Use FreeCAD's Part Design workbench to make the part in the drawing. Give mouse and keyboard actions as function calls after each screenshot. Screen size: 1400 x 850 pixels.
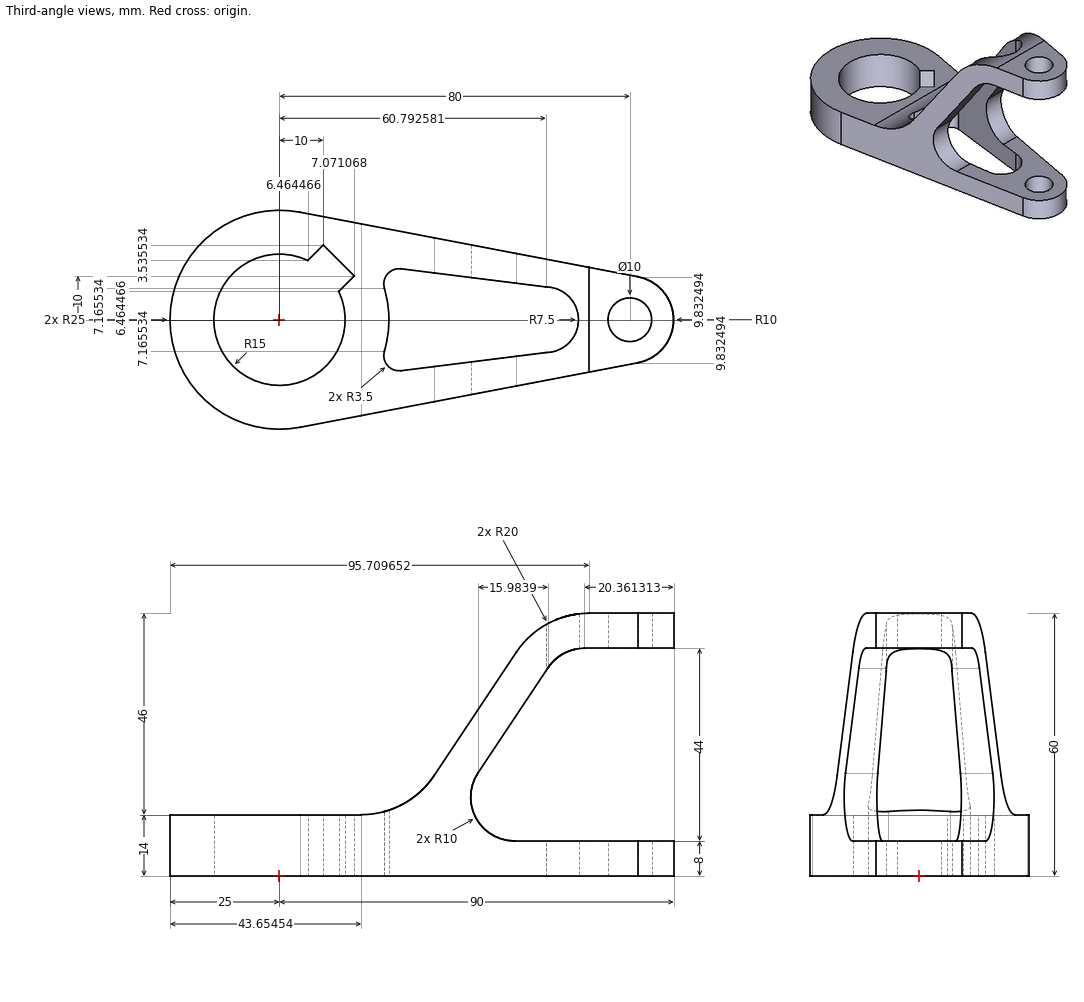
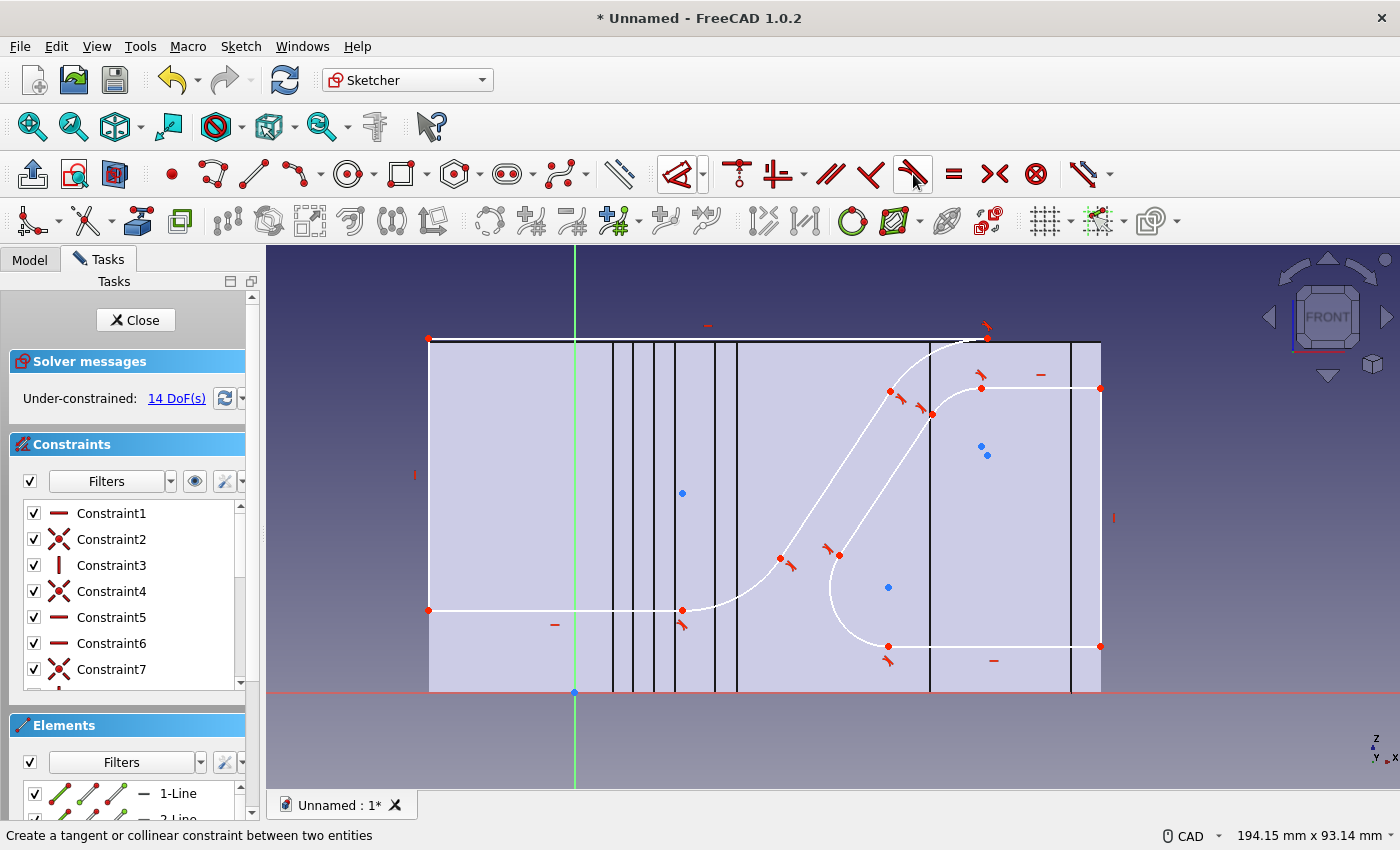
click(914, 366)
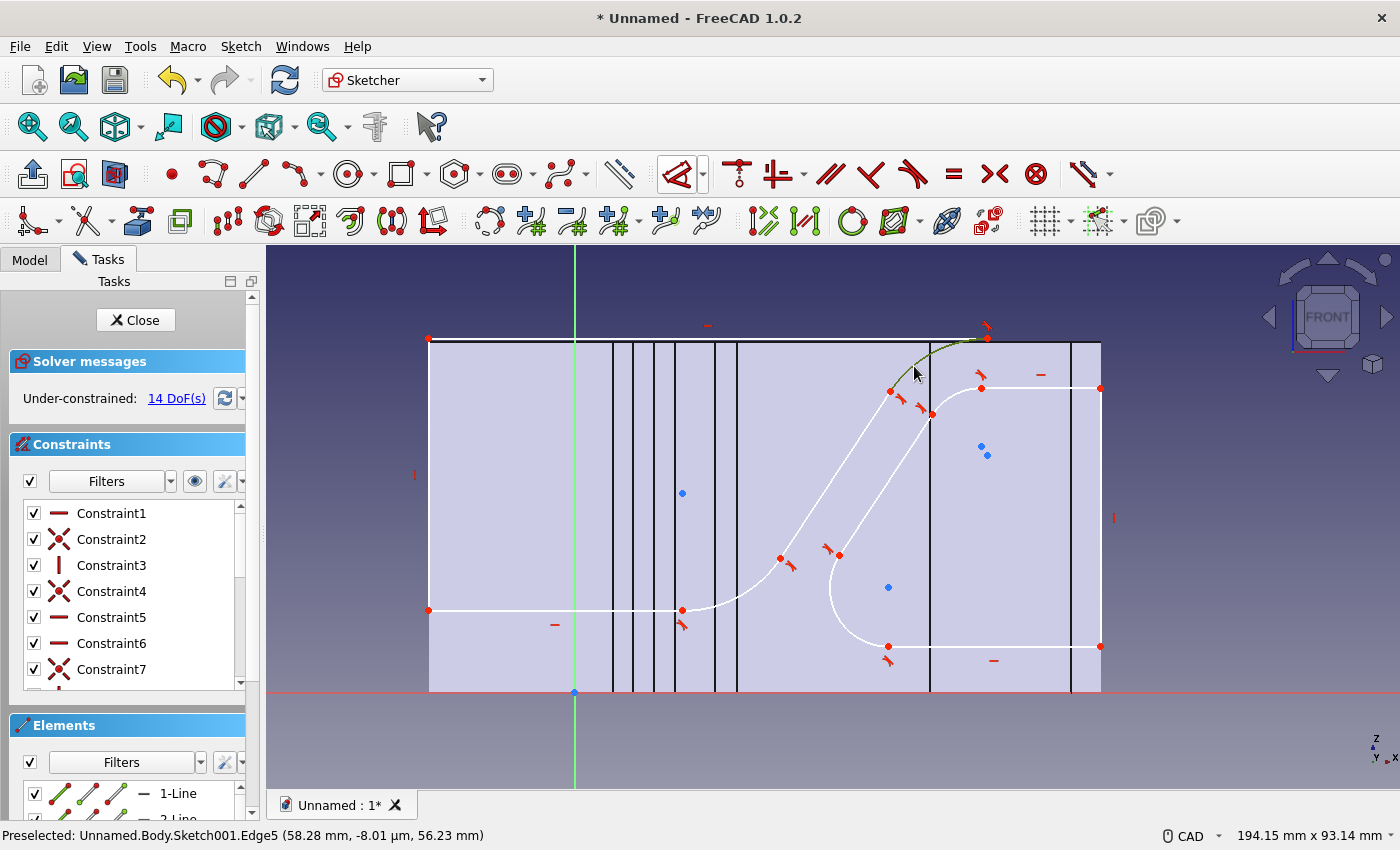
click(717, 606)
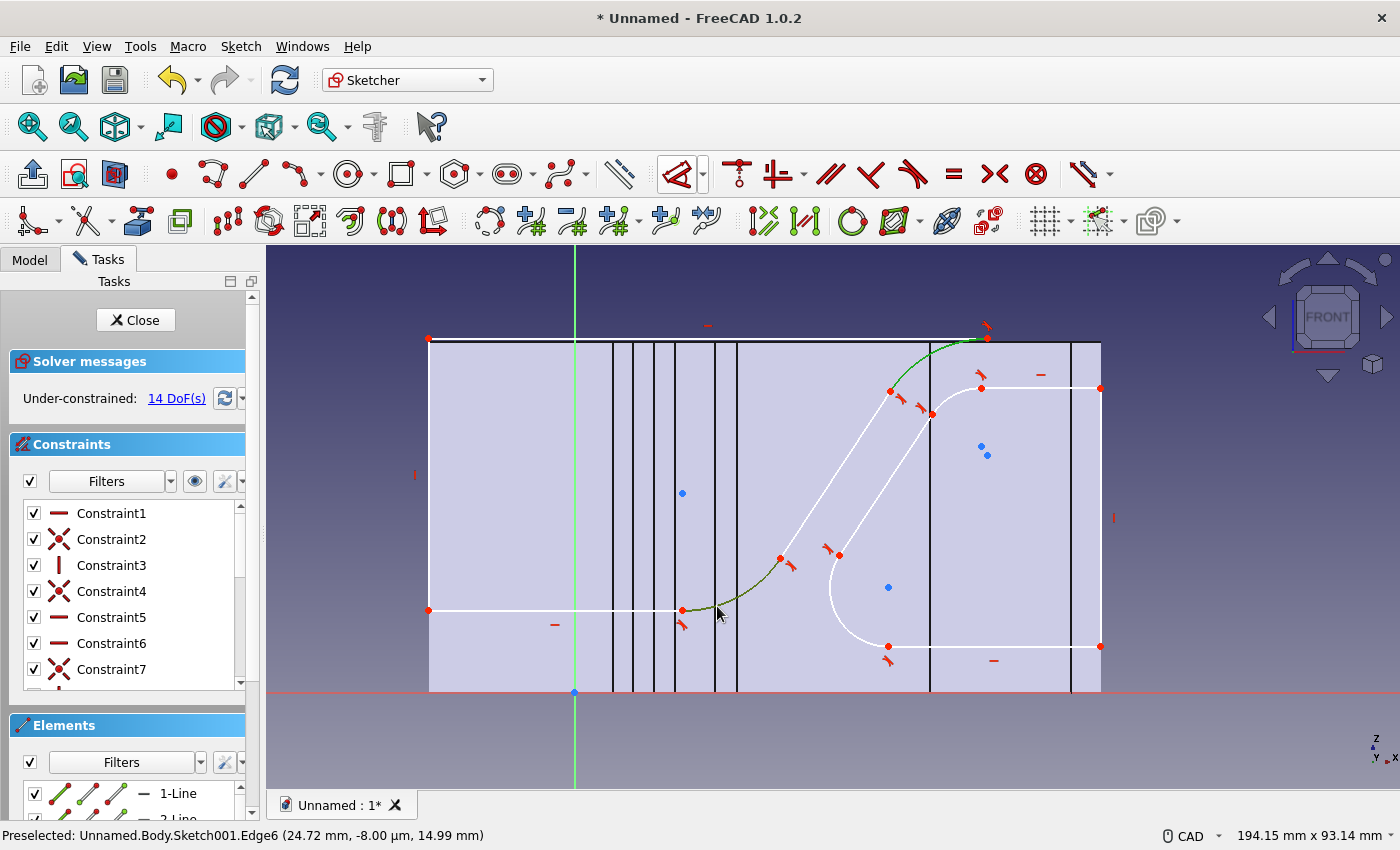
click(954, 174)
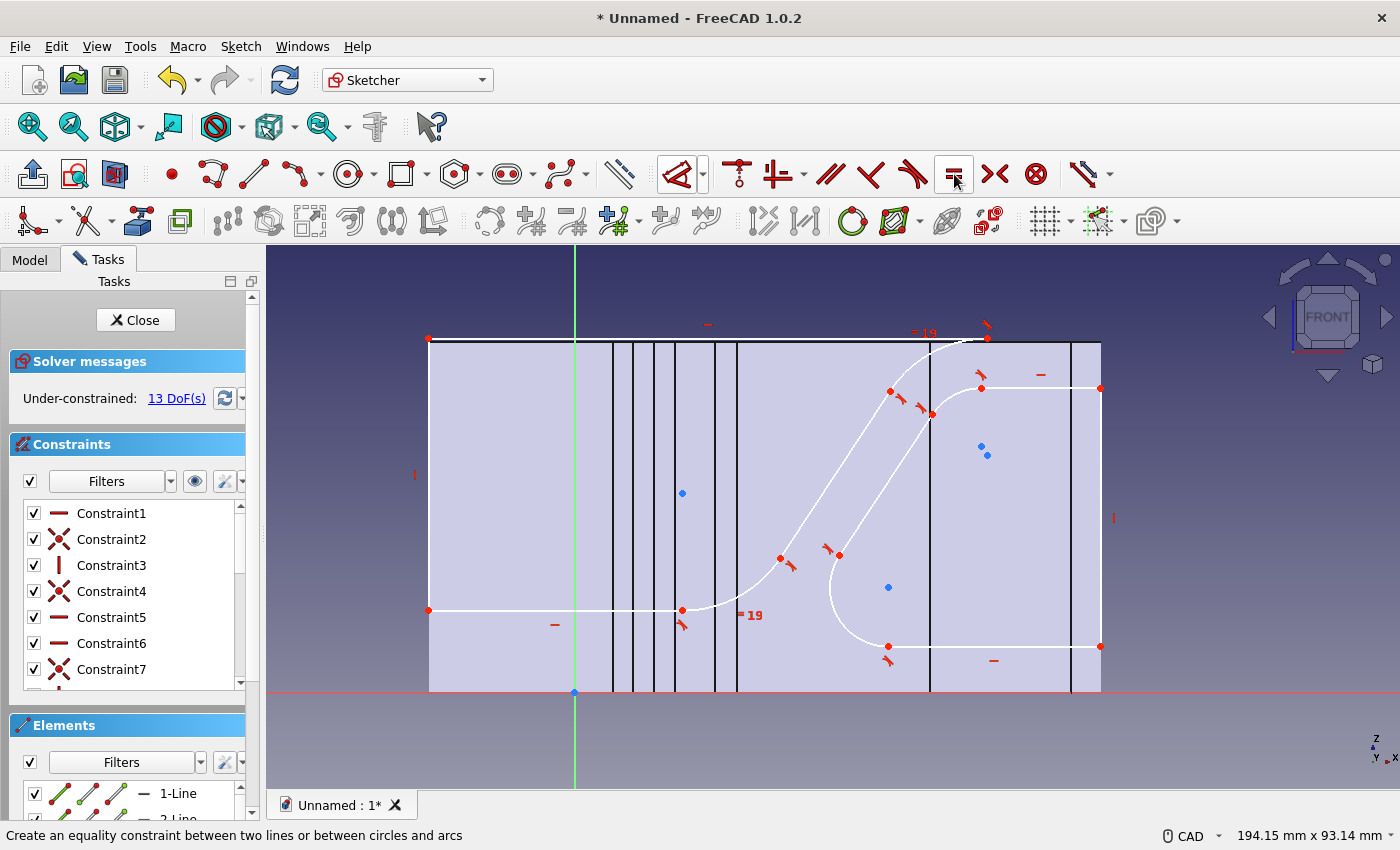
click(964, 391)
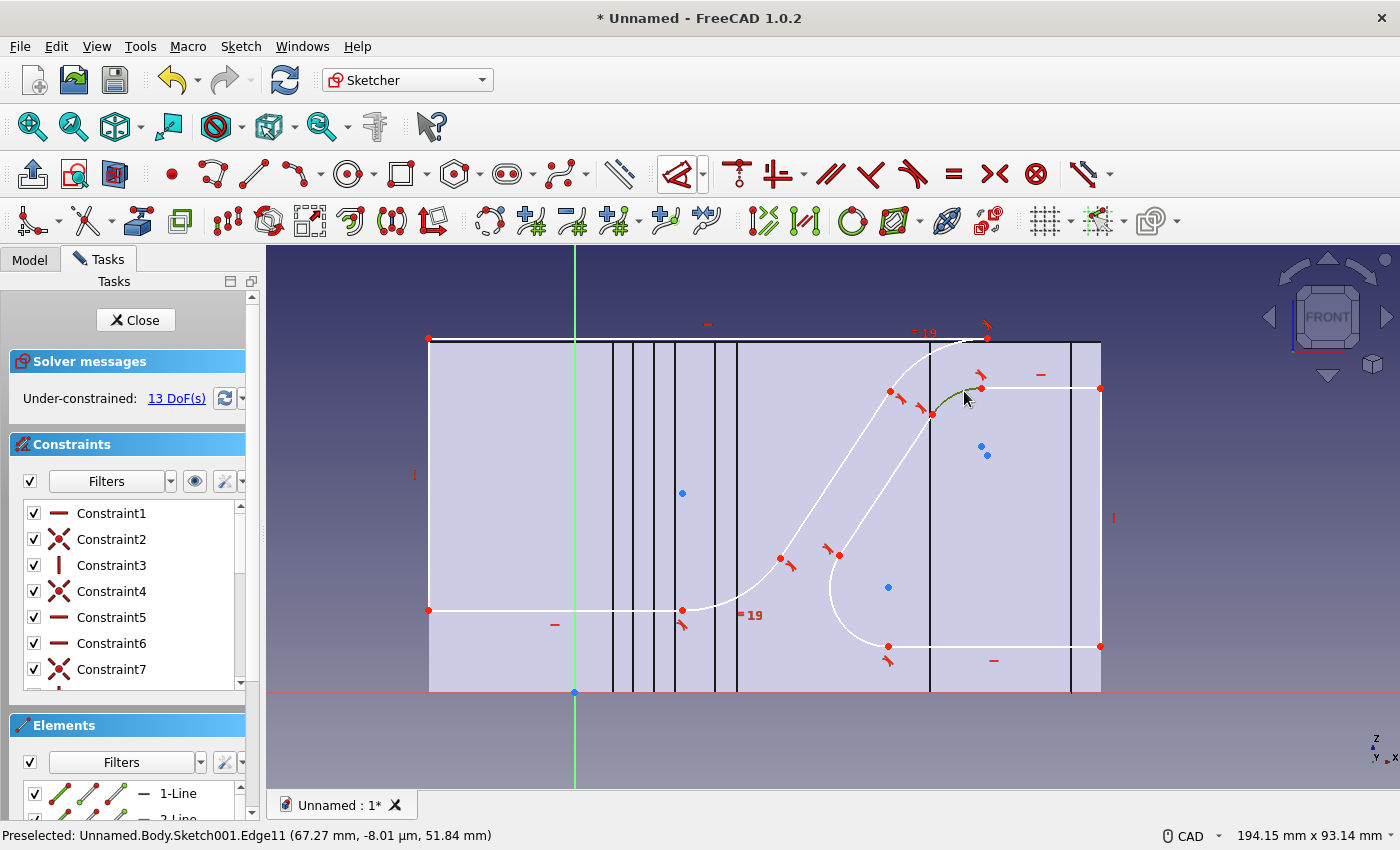
click(830, 592)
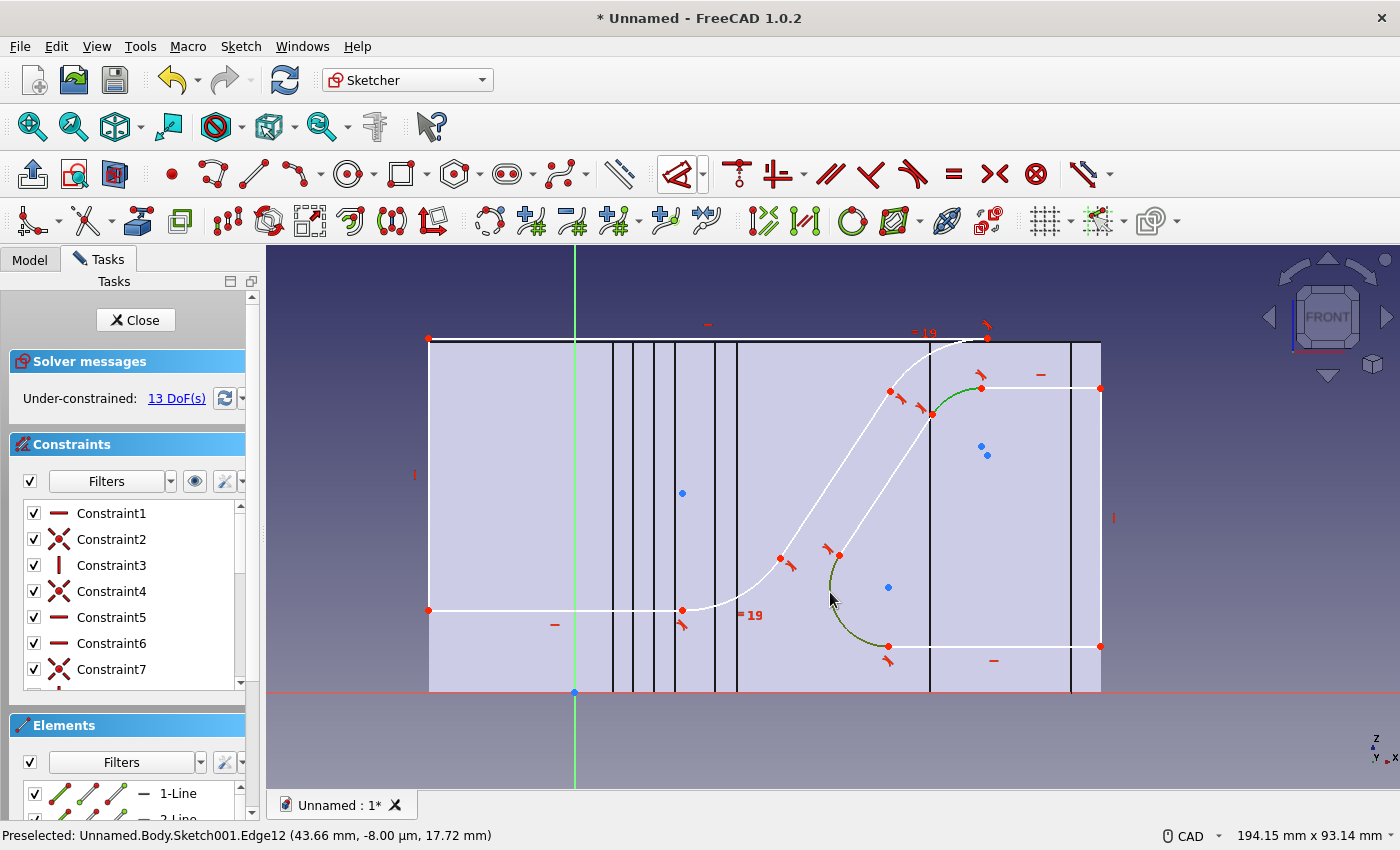
click(954, 174)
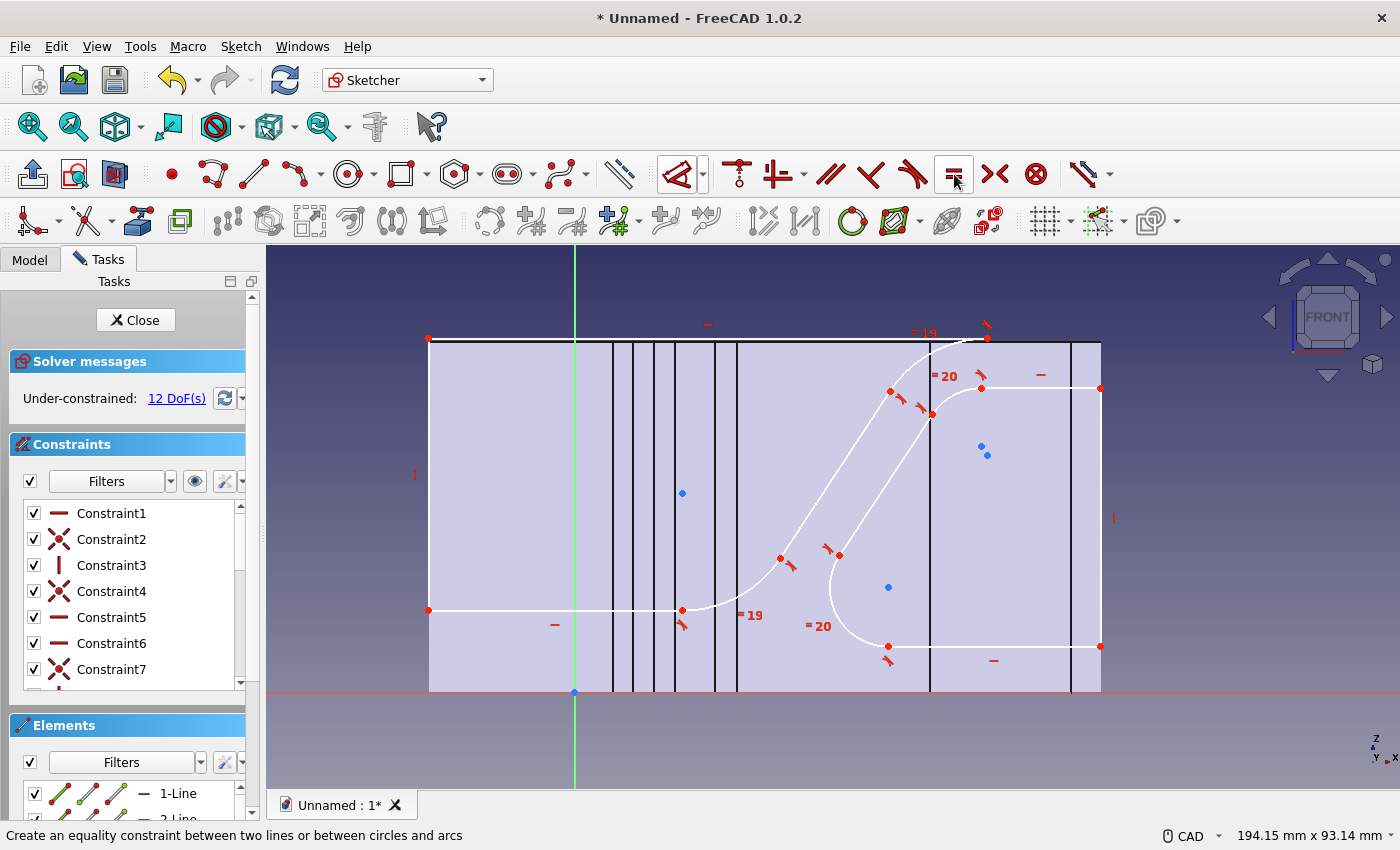
click(913, 365)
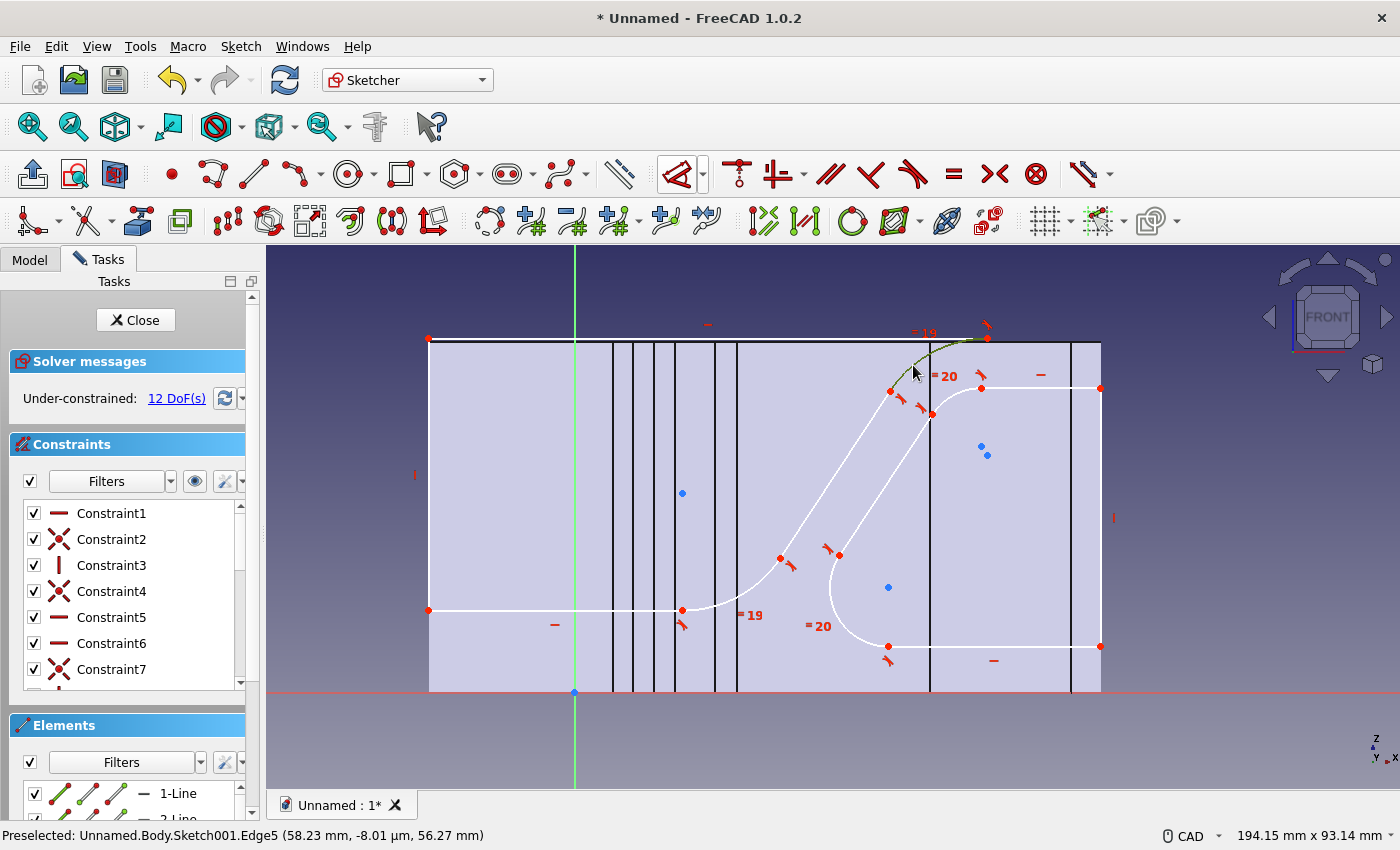
click(702, 174)